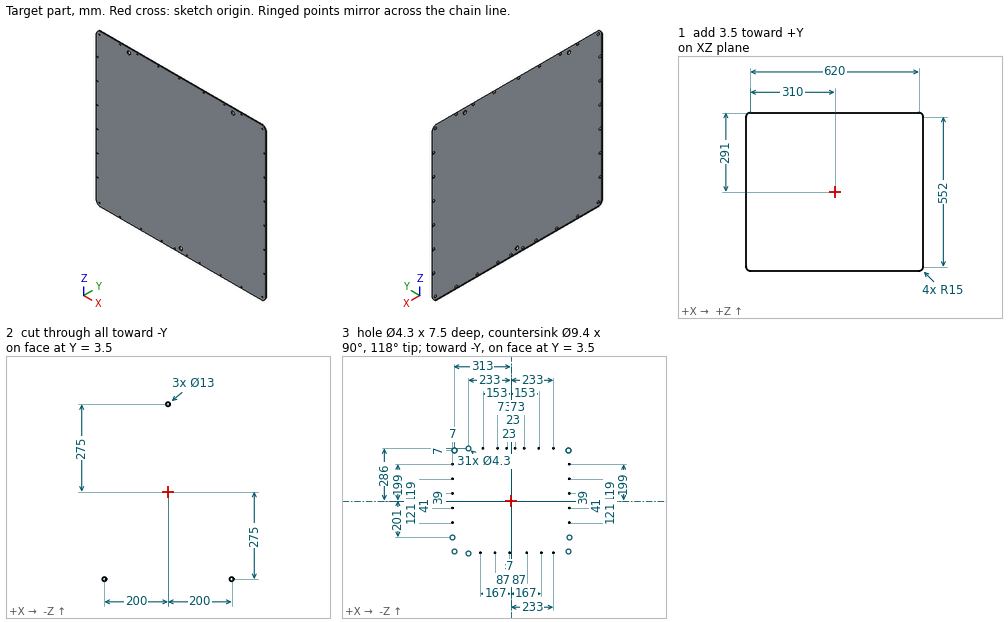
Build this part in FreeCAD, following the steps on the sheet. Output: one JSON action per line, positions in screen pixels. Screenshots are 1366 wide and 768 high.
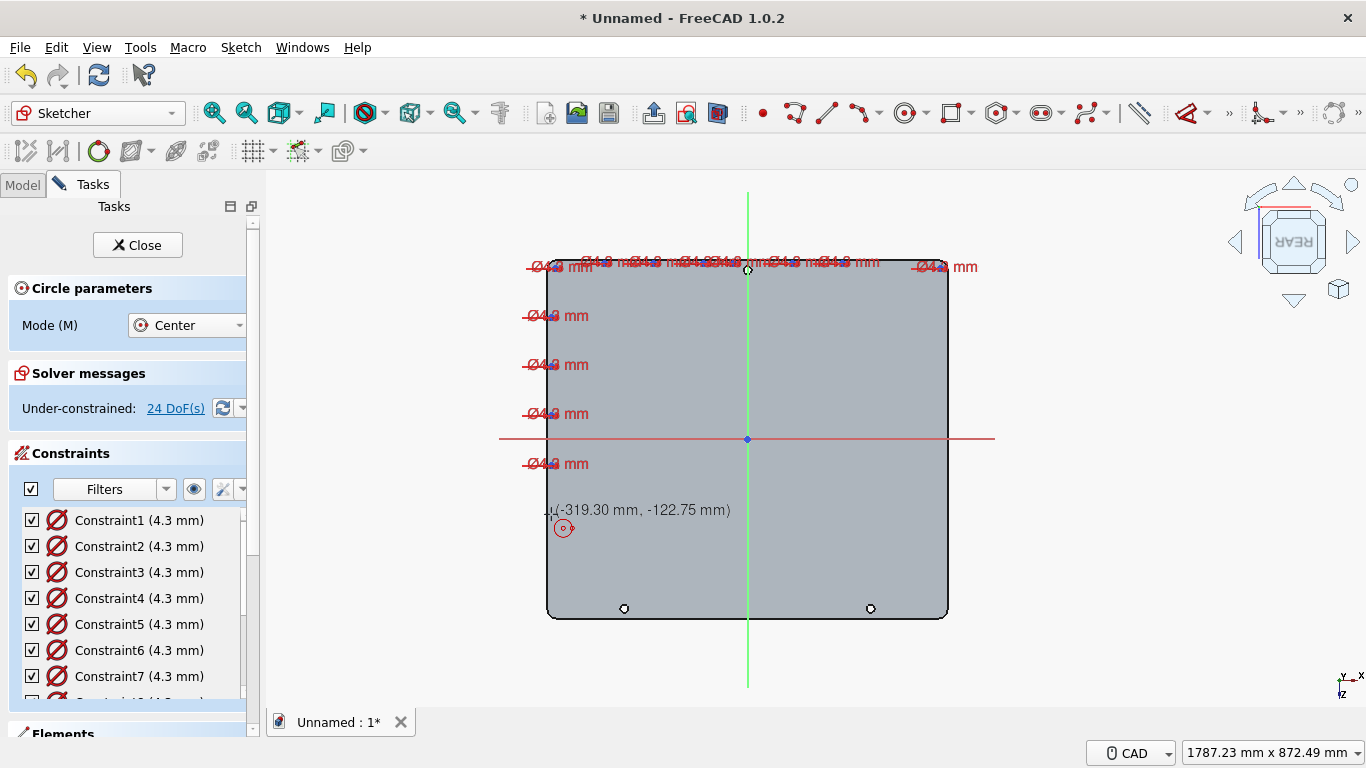
{"action": "left_click", "coordinate": [551, 514]}
{"action": "mouse_move", "coordinate": [552, 513]}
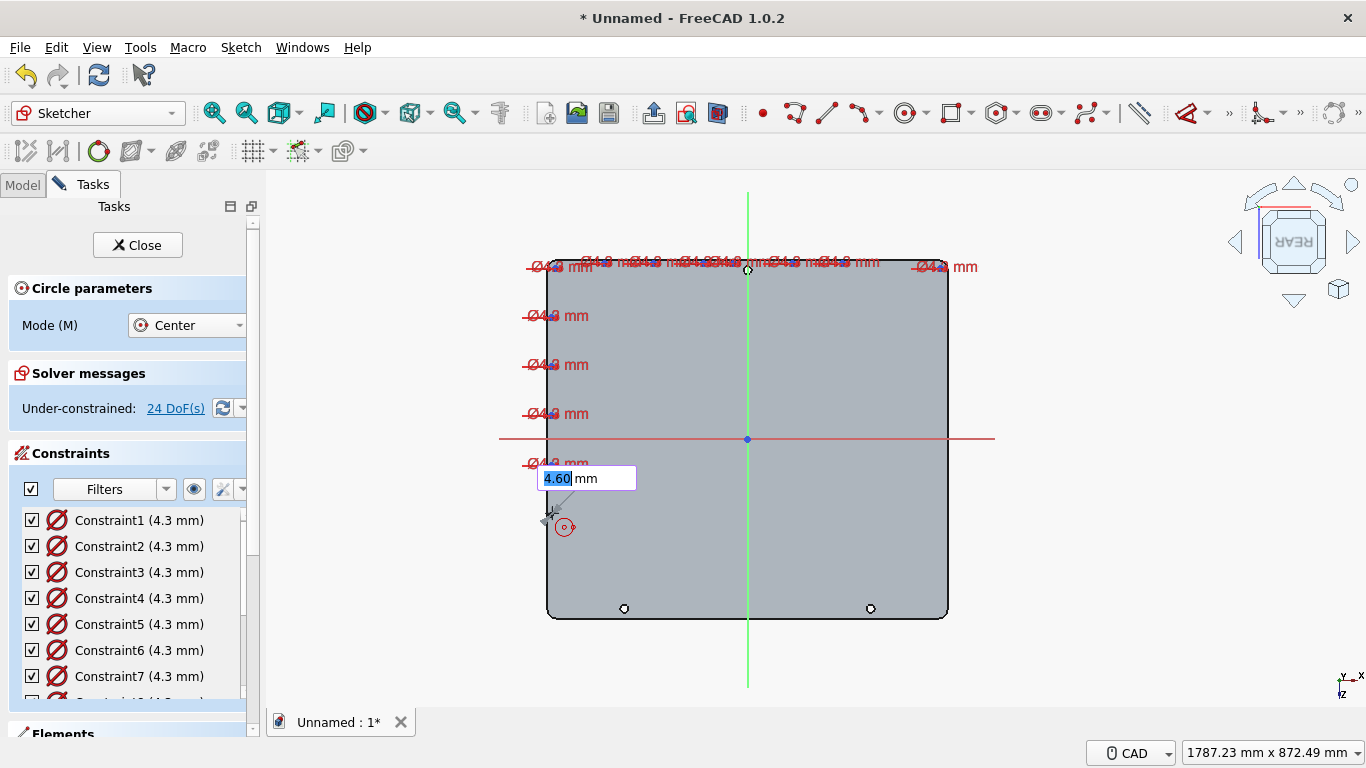
{"action": "type", "text": "4.3"}
{"action": "key", "text": "Return"}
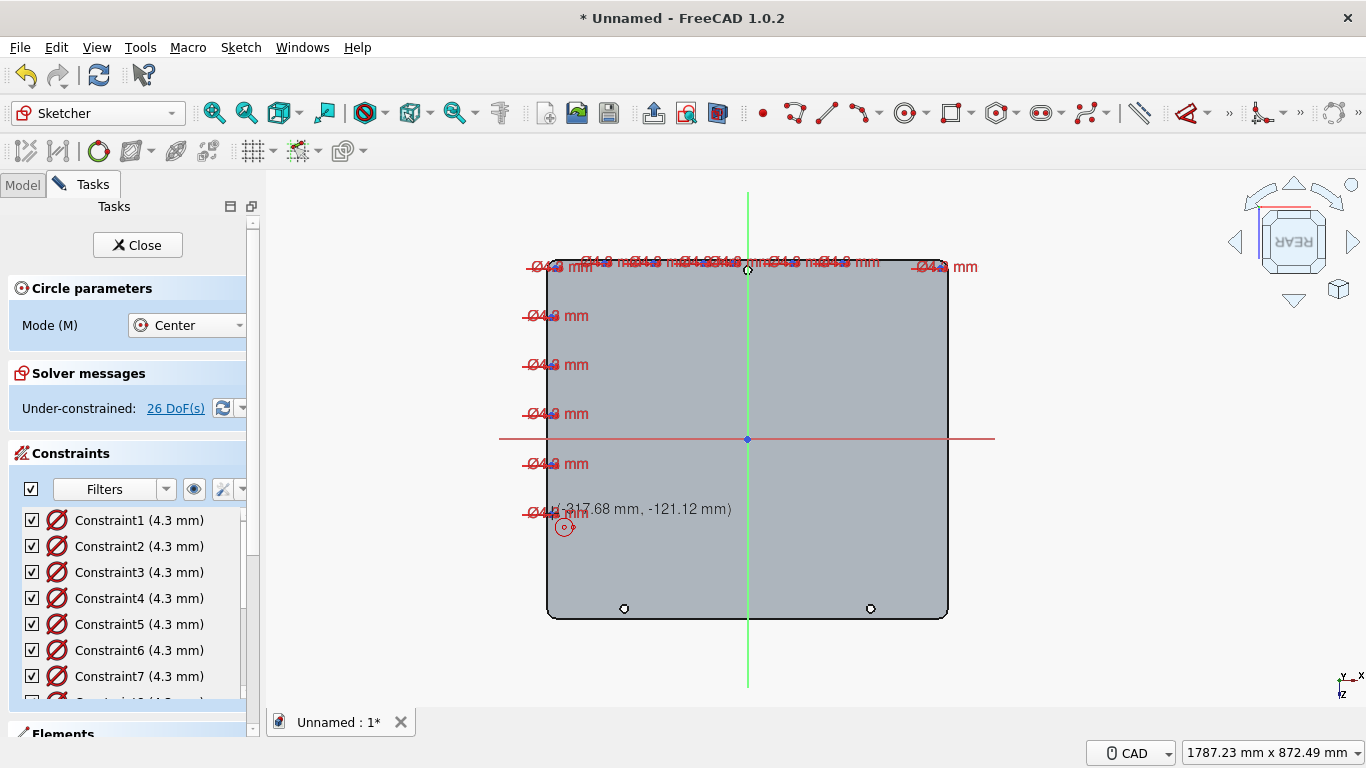
{"action": "scroll", "coordinate": [551, 563], "scroll_direction": "up", "scroll_amount": 15}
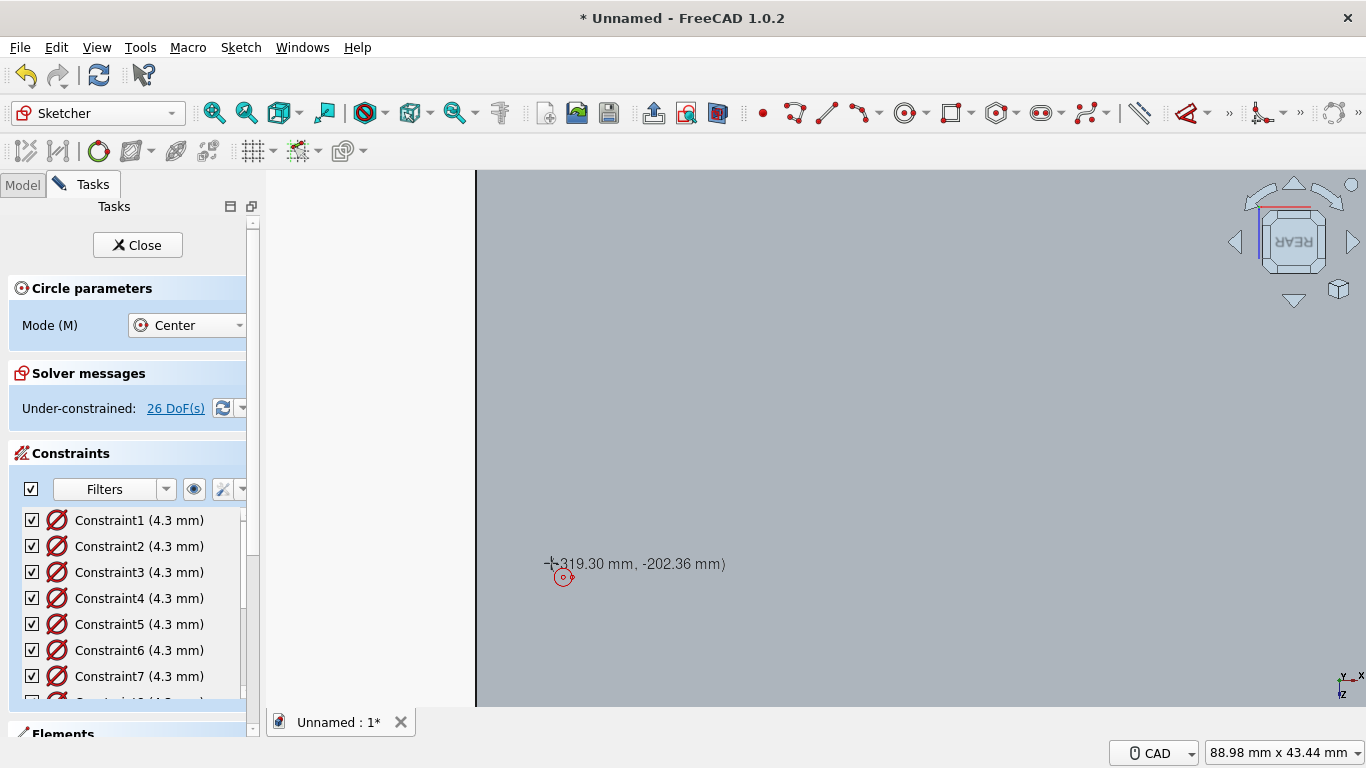
{"action": "scroll", "coordinate": [551, 563], "scroll_direction": "down", "scroll_amount": 15}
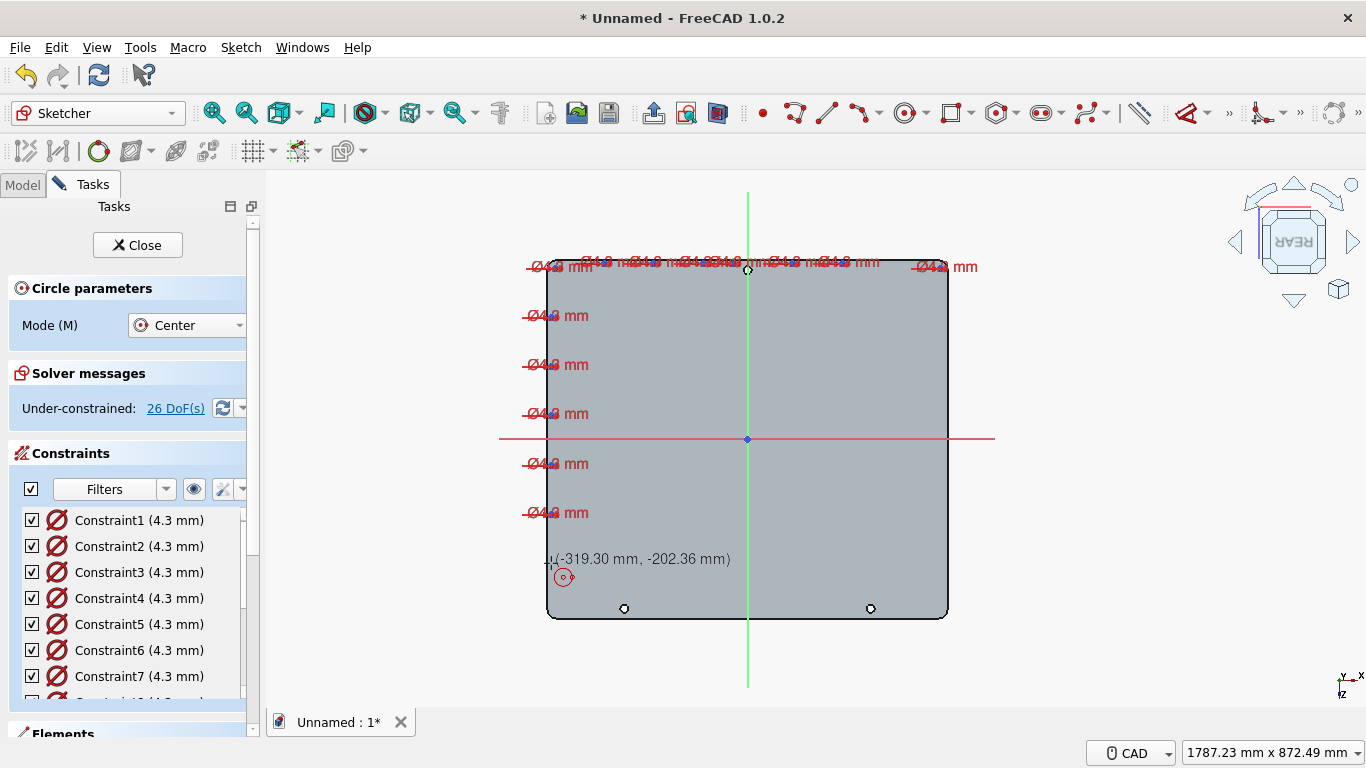
{"action": "left_click", "coordinate": [551, 563]}
{"action": "mouse_move", "coordinate": [552, 562]}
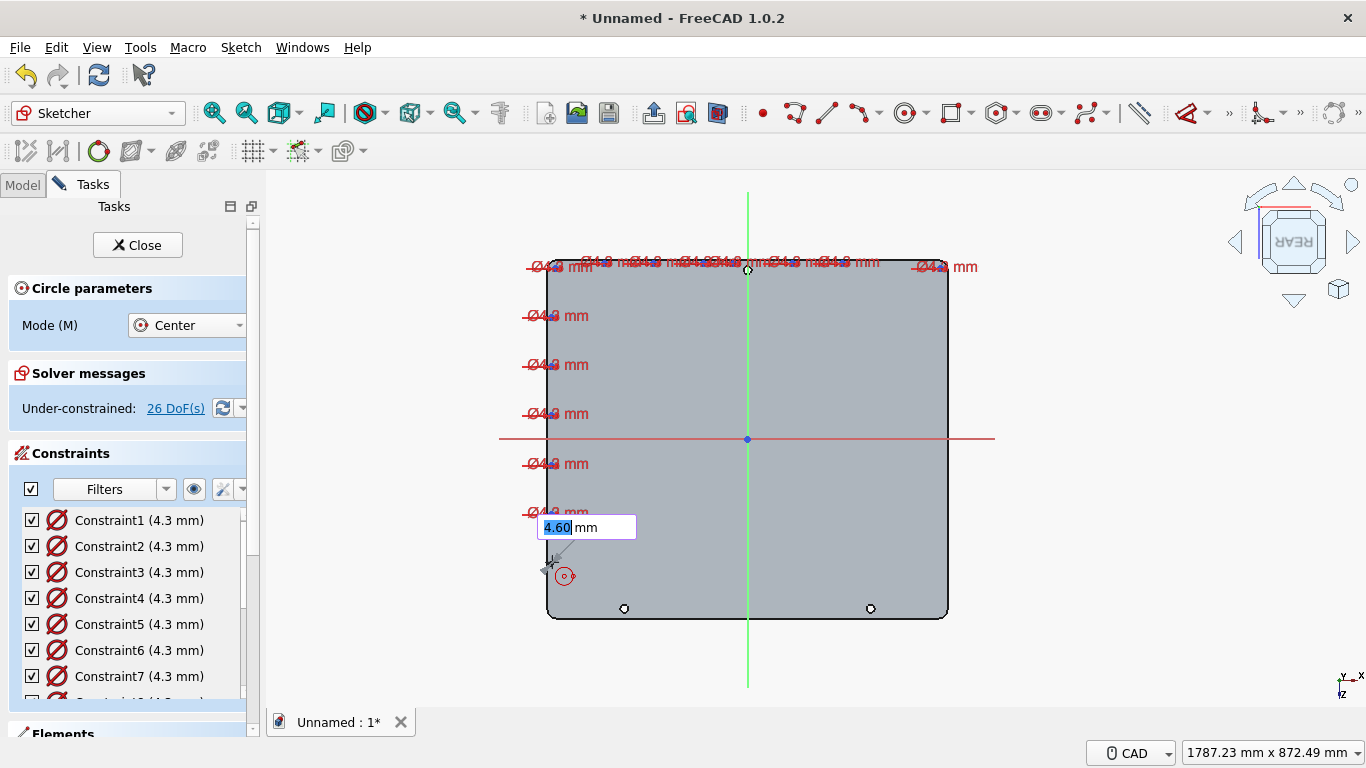
{"action": "type", "text": "4.3"}
{"action": "key", "text": "Return"}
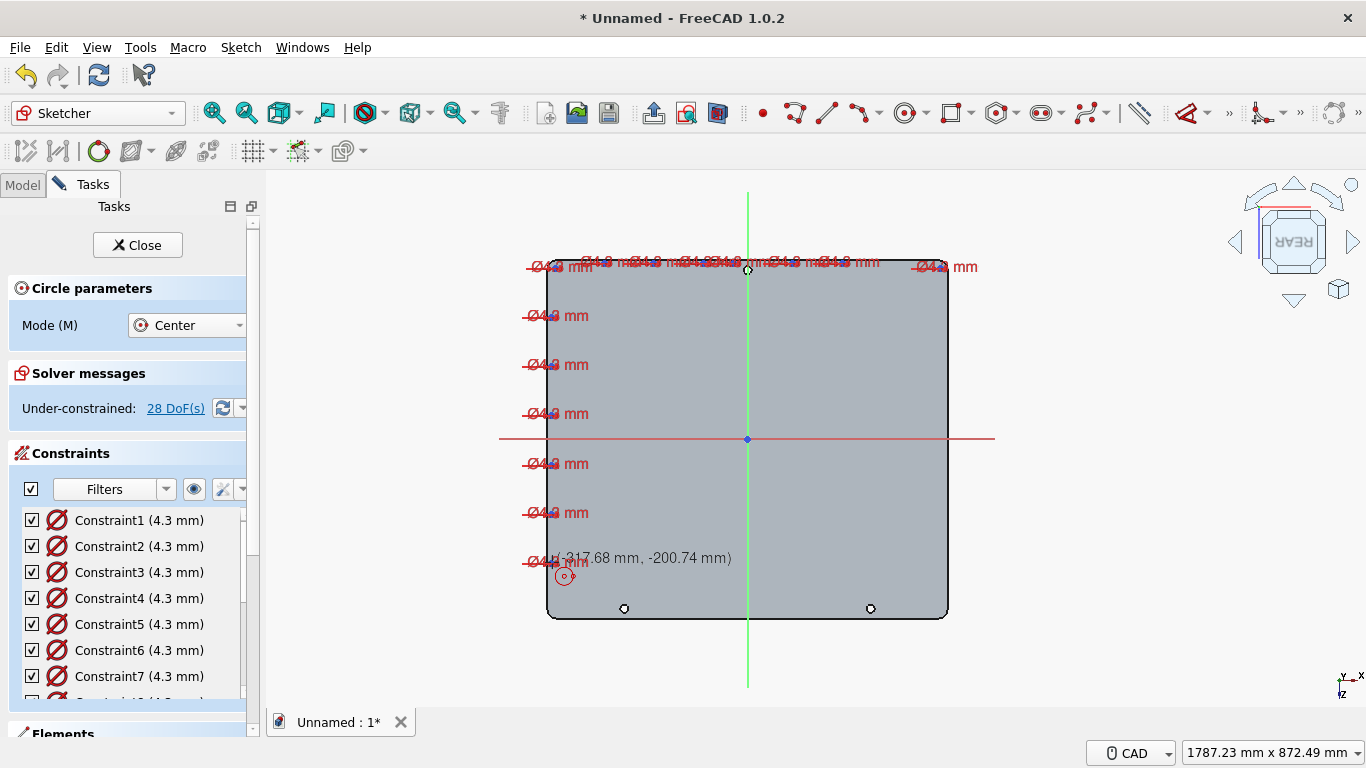
{"action": "scroll", "coordinate": [555, 611], "scroll_direction": "up", "scroll_amount": 15}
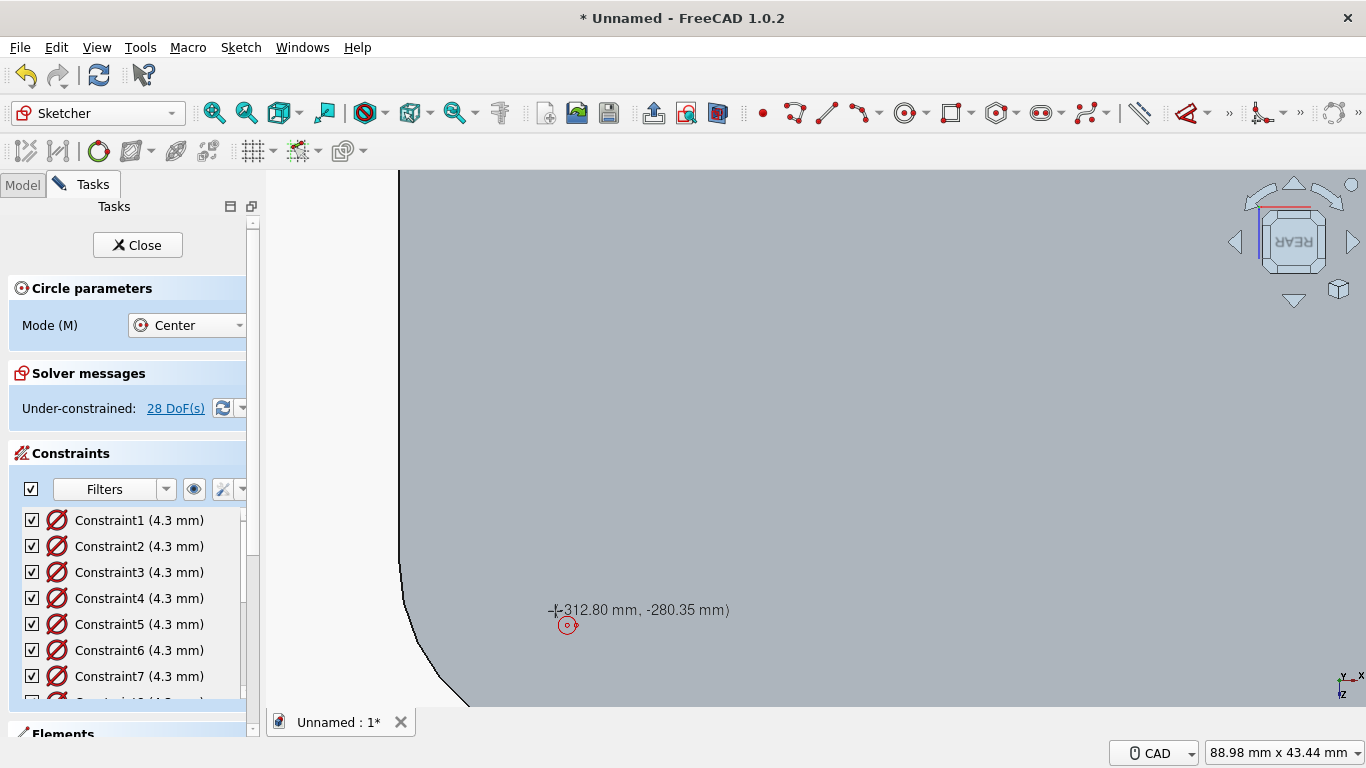
{"action": "scroll", "coordinate": [555, 611], "scroll_direction": "down", "scroll_amount": 15}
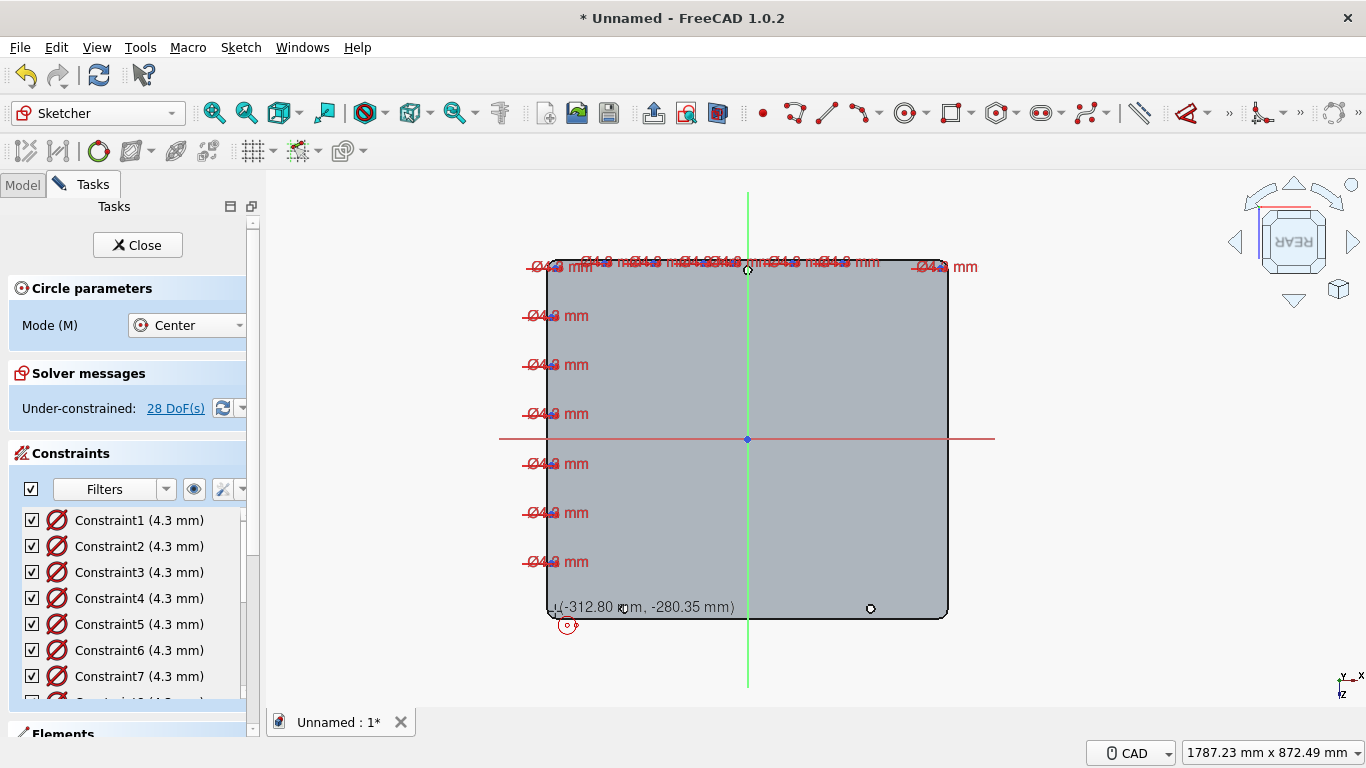
{"action": "left_click", "coordinate": [555, 611]}
{"action": "mouse_move", "coordinate": [556, 610]}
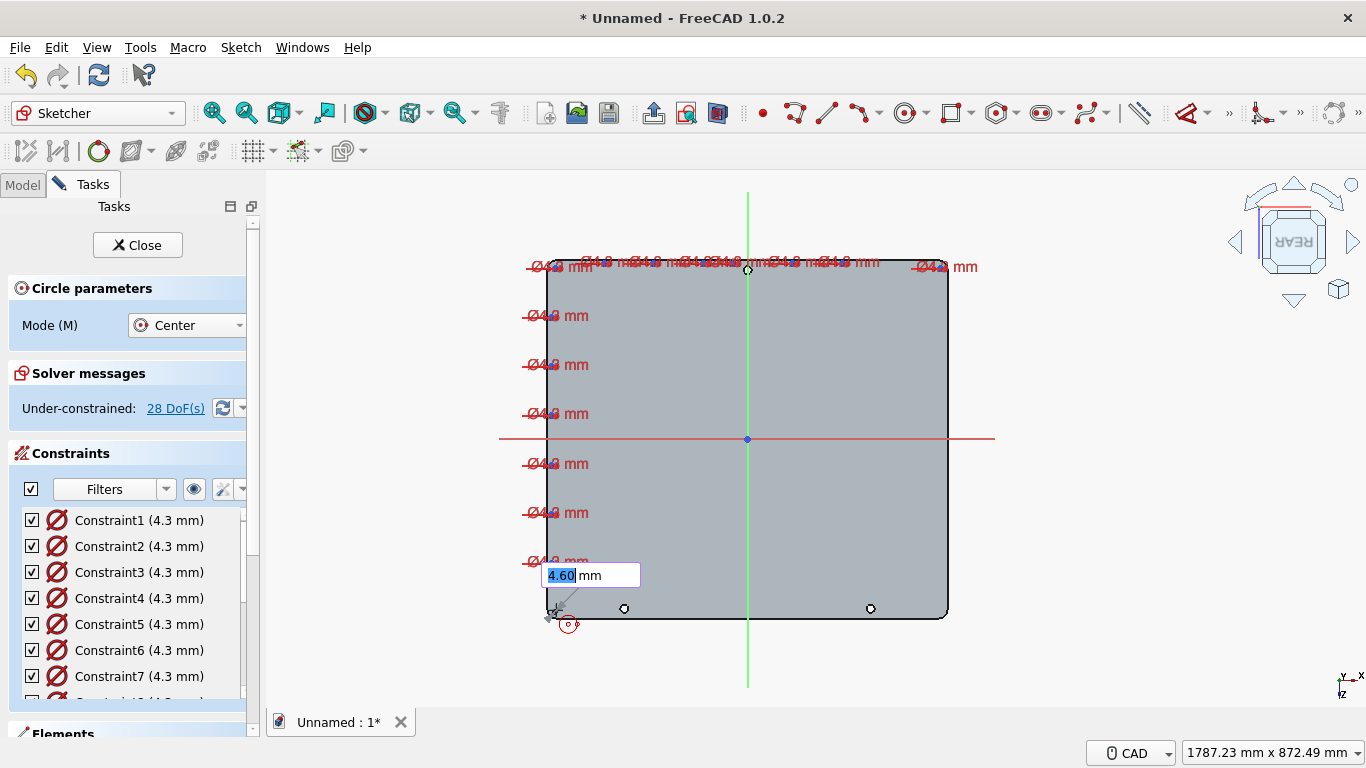
{"action": "type", "text": "4.3"}
{"action": "key", "text": "Return"}